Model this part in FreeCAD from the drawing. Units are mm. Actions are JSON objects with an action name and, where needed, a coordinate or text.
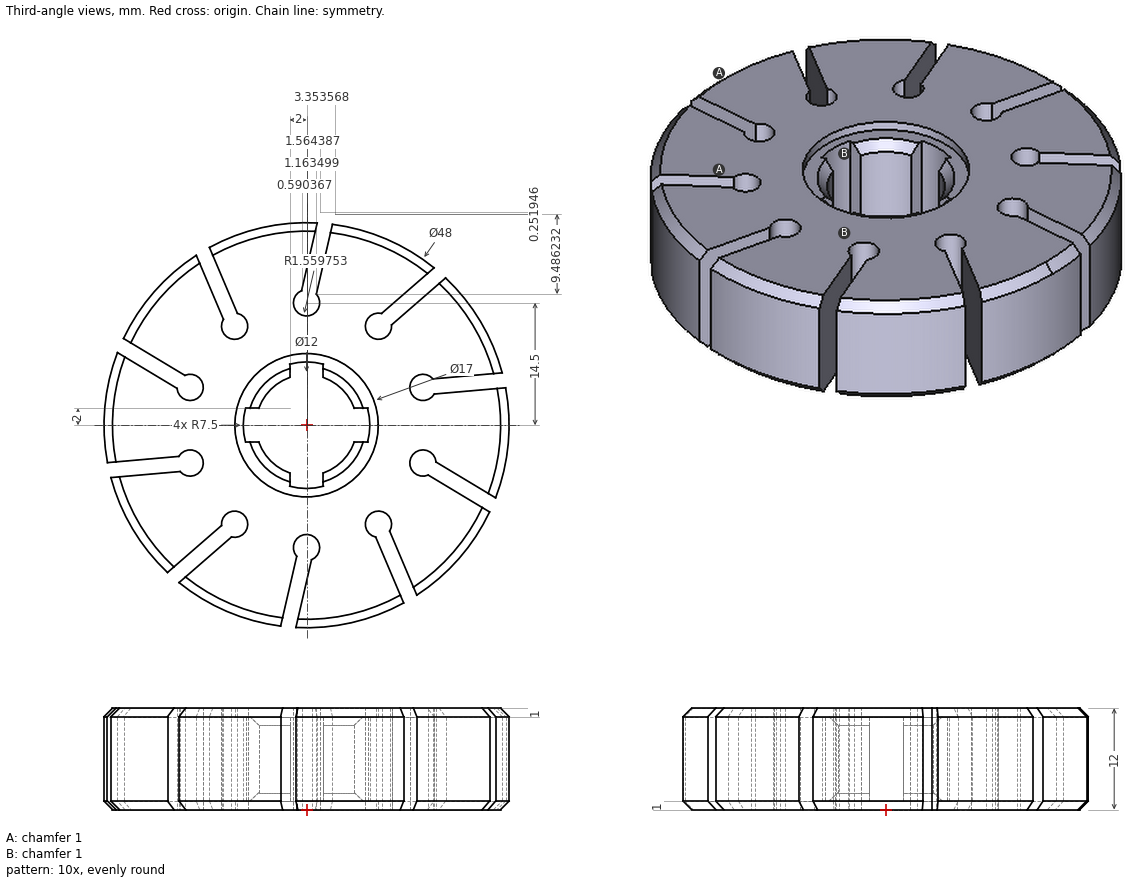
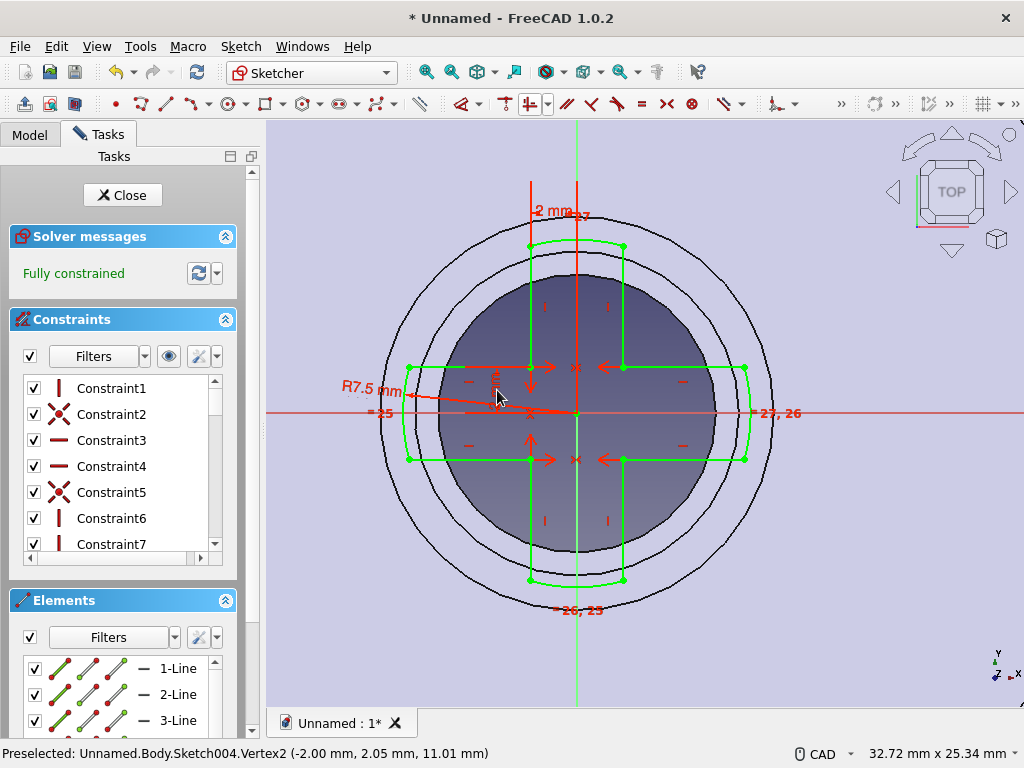
{"action": "left_click", "coordinate": [123, 195]}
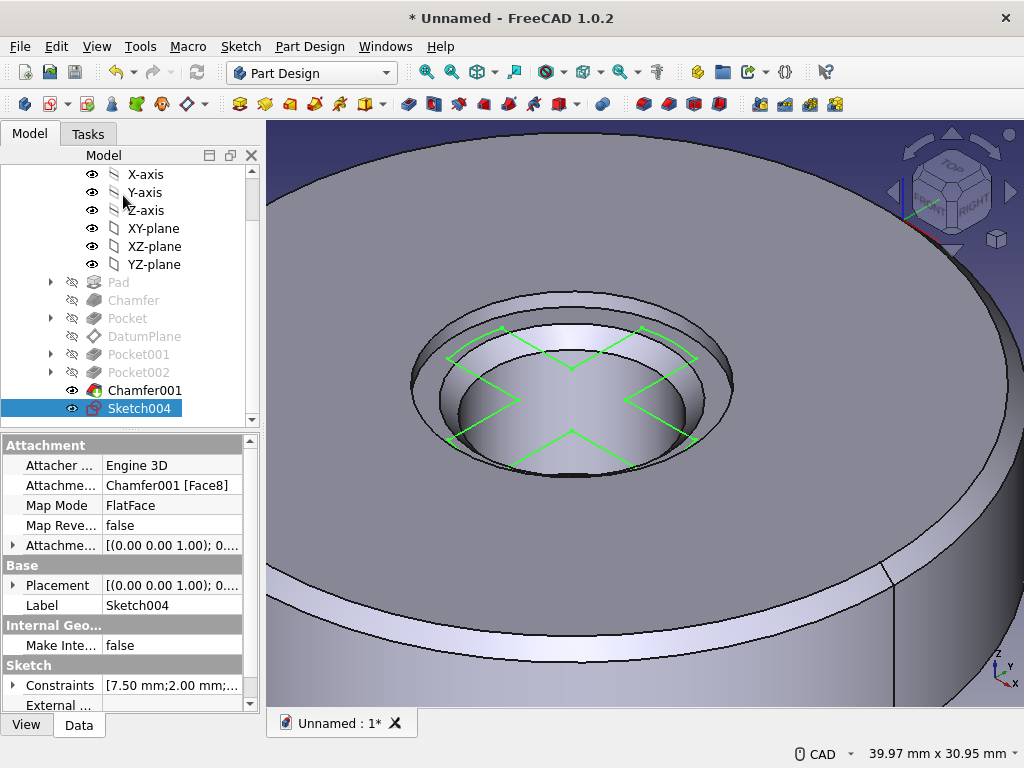
{"action": "left_click", "coordinate": [409, 104]}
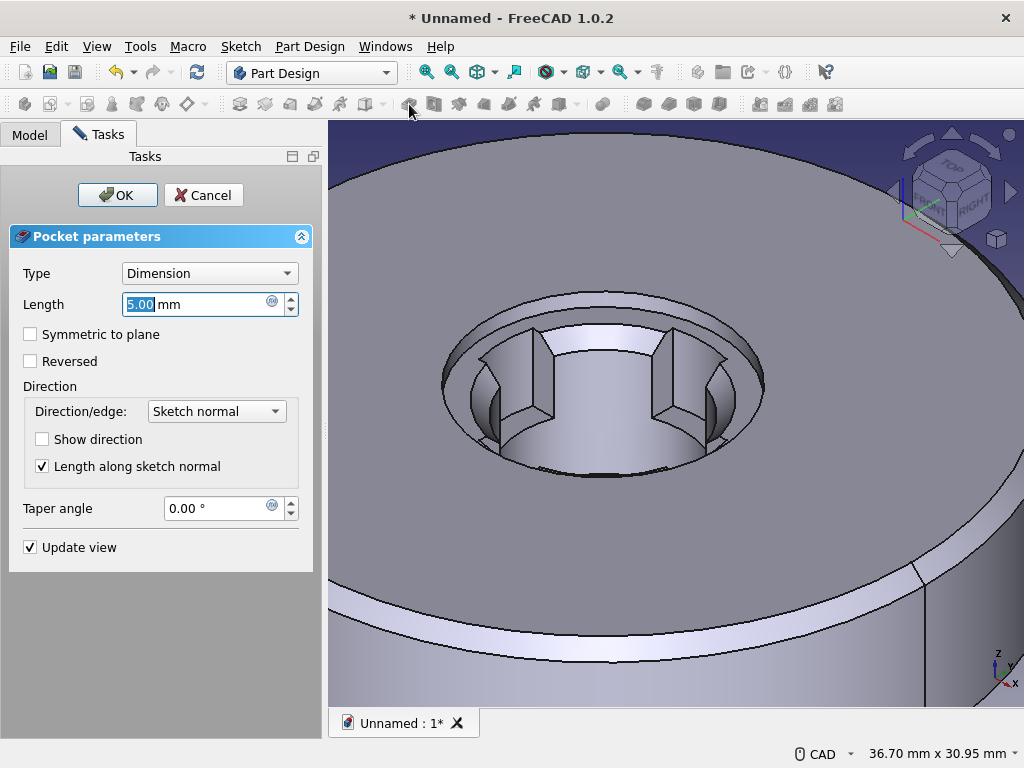
{"action": "left_click", "coordinate": [210, 274]}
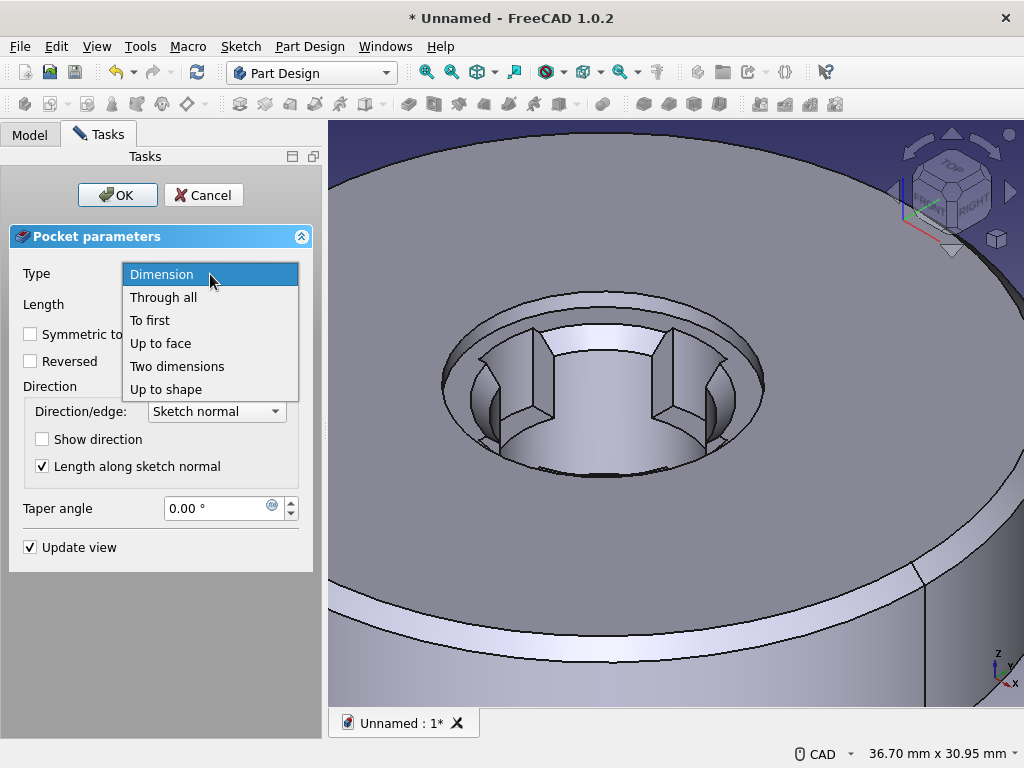
{"action": "left_click", "coordinate": [208, 298]}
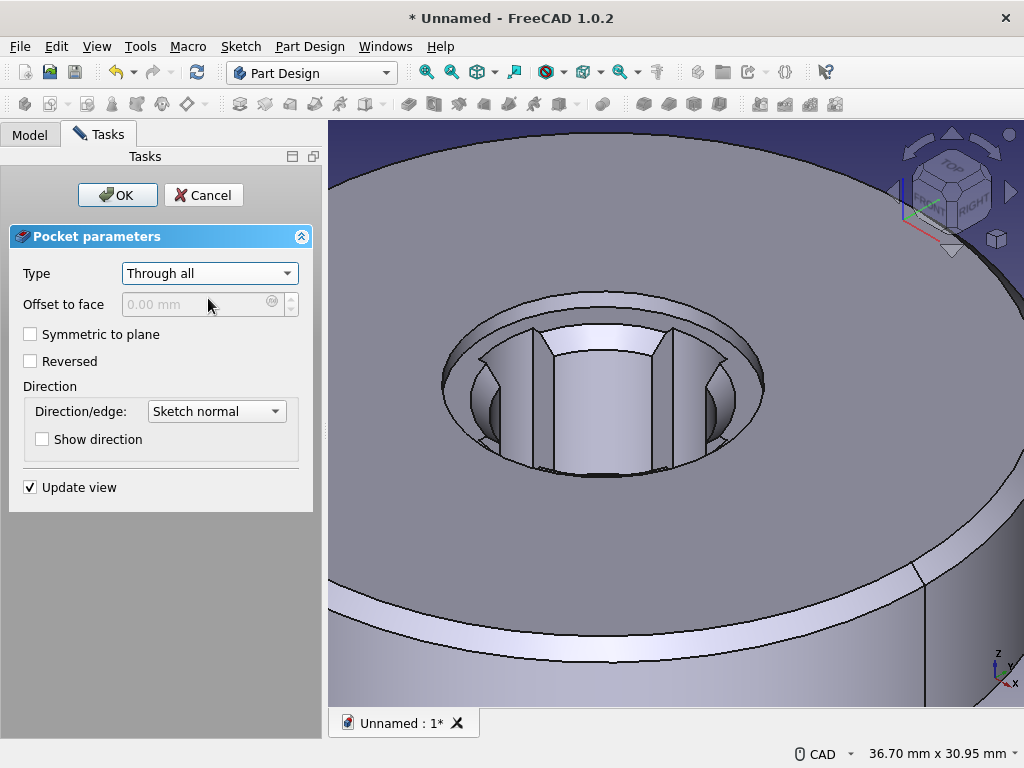
{"action": "left_click", "coordinate": [118, 195]}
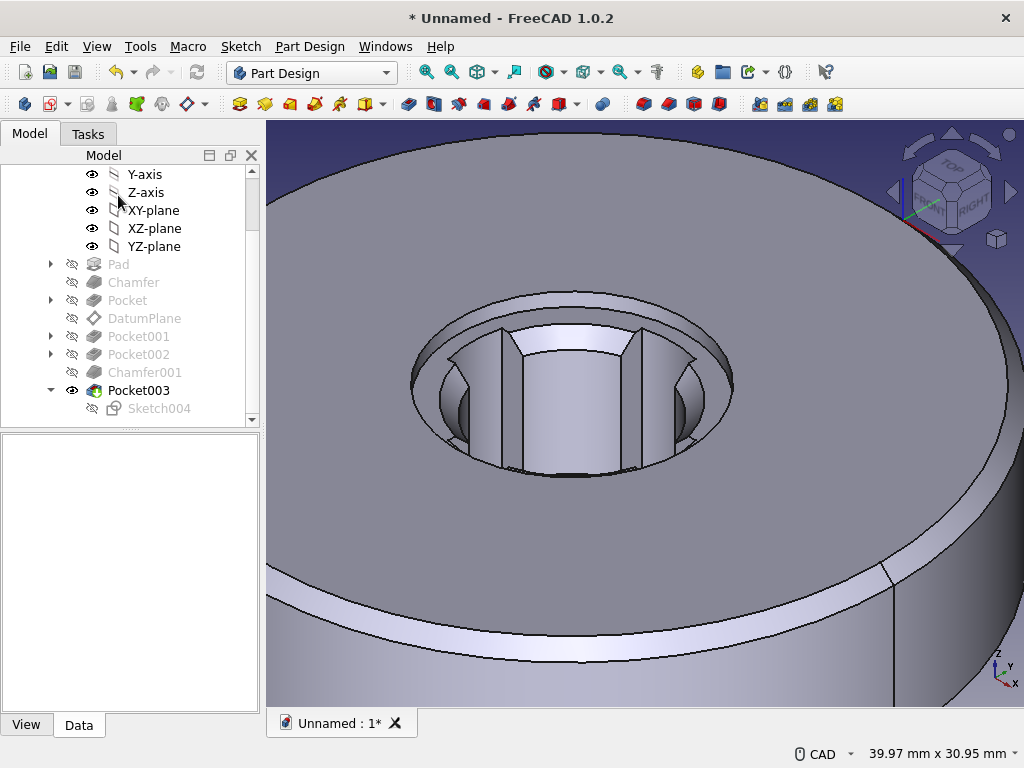
{"action": "left_click", "coordinate": [427, 72]}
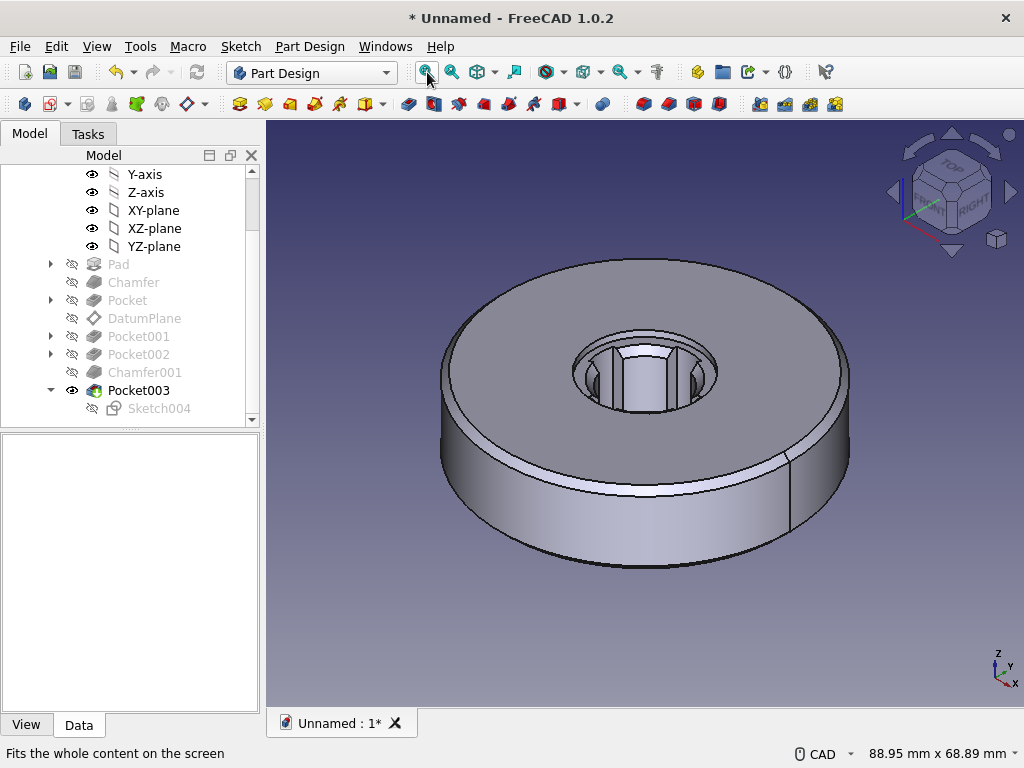
{"action": "left_click", "coordinate": [685, 302]}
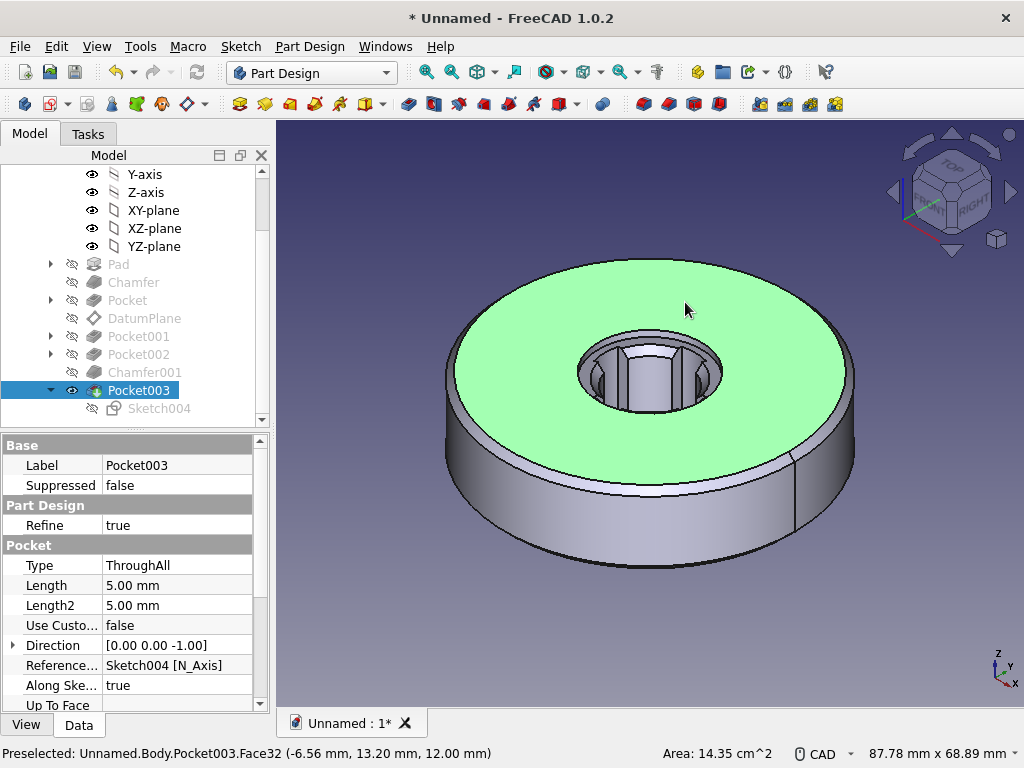
{"action": "left_click", "coordinate": [50, 104]}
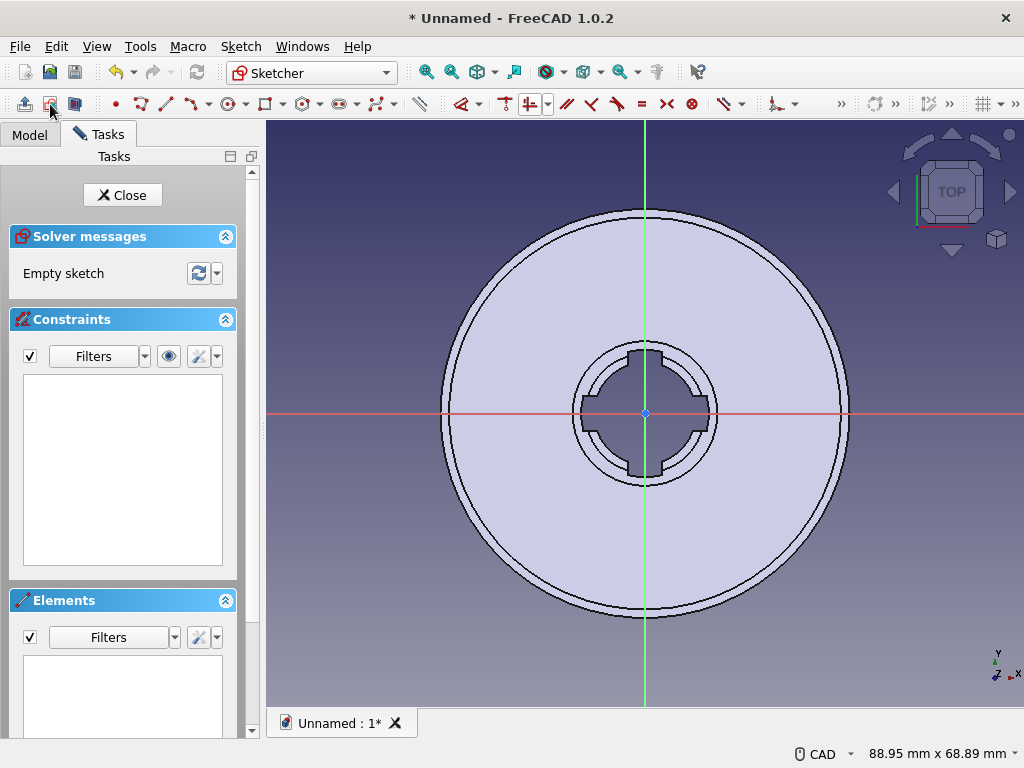
{"action": "scroll", "coordinate": [754, 175], "scroll_direction": "up", "scroll_amount": 3}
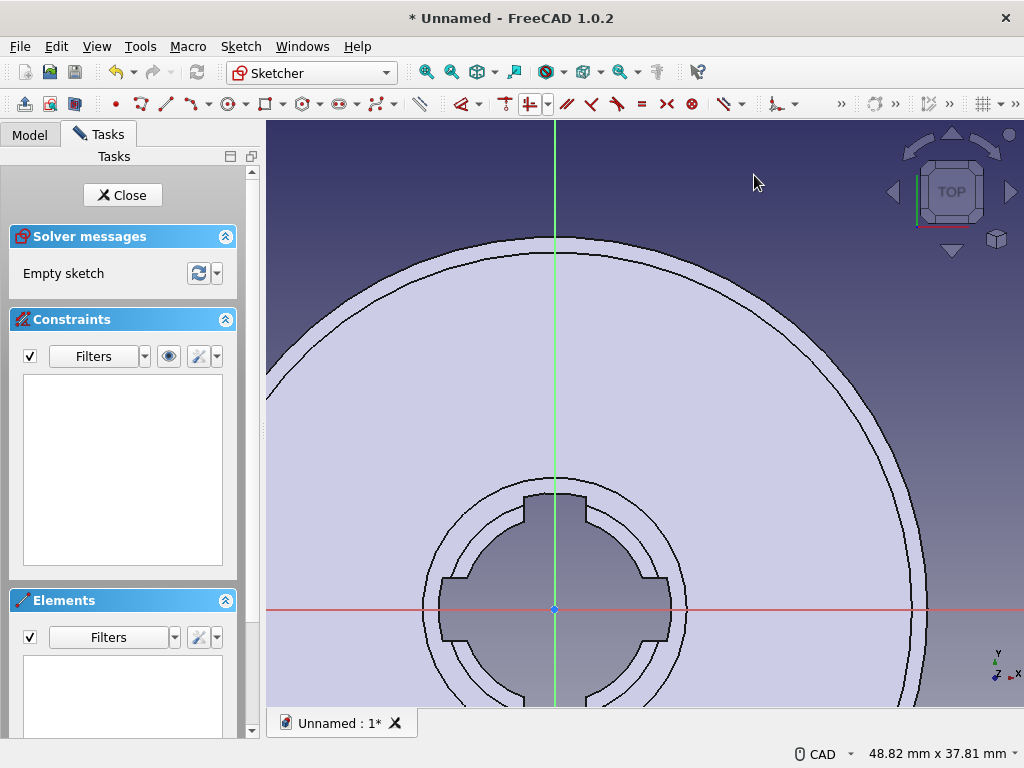
{"action": "left_click", "coordinate": [141, 104]}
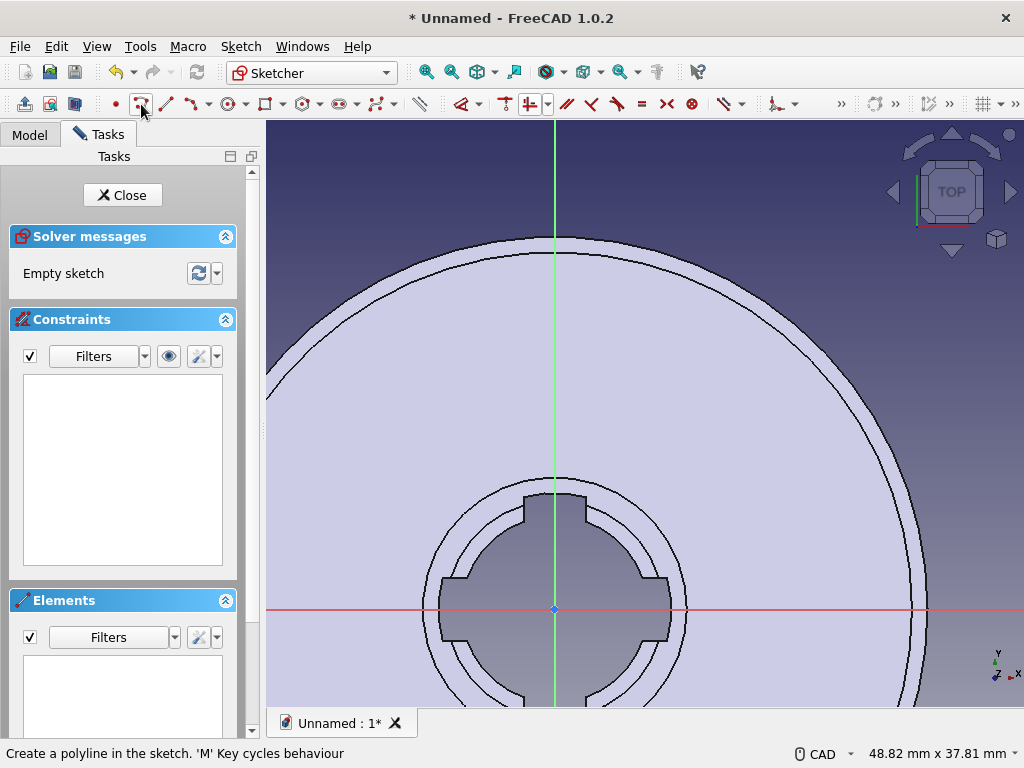
{"action": "left_click", "coordinate": [573, 368]}
{"action": "left_click", "coordinate": [607, 221]}
{"action": "left_click", "coordinate": [579, 217]}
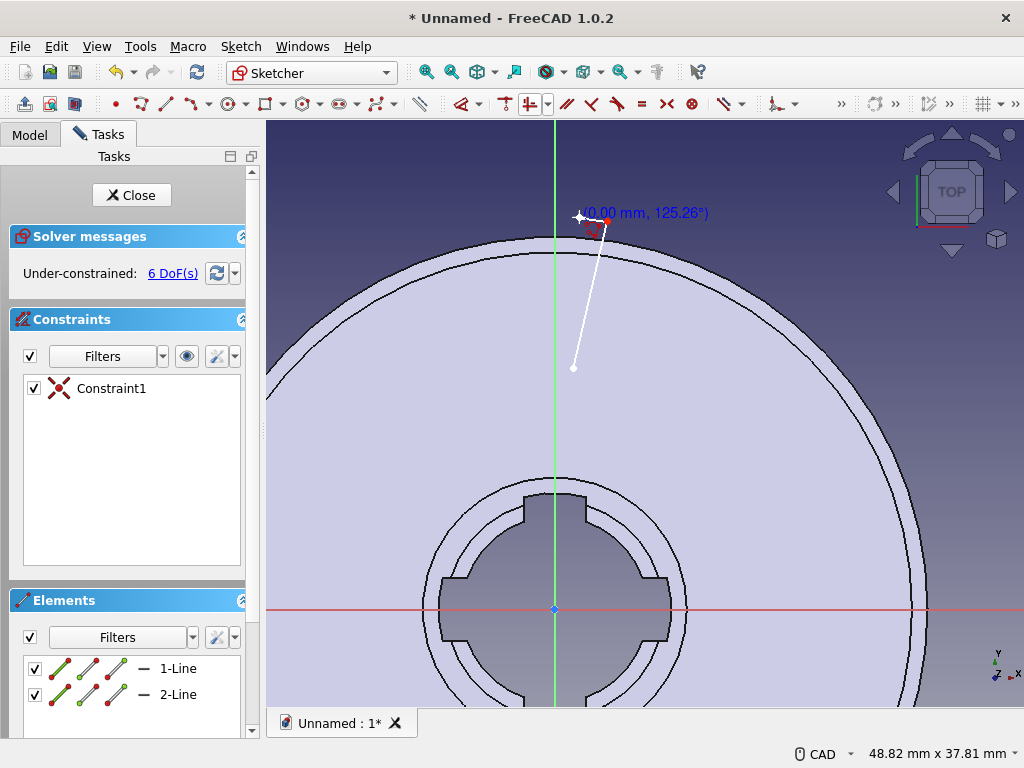
{"action": "scroll", "coordinate": [546, 362], "scroll_direction": "up", "scroll_amount": 3}